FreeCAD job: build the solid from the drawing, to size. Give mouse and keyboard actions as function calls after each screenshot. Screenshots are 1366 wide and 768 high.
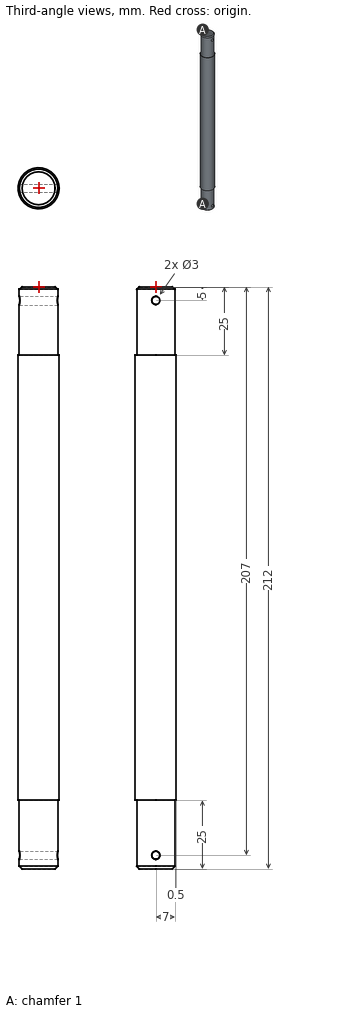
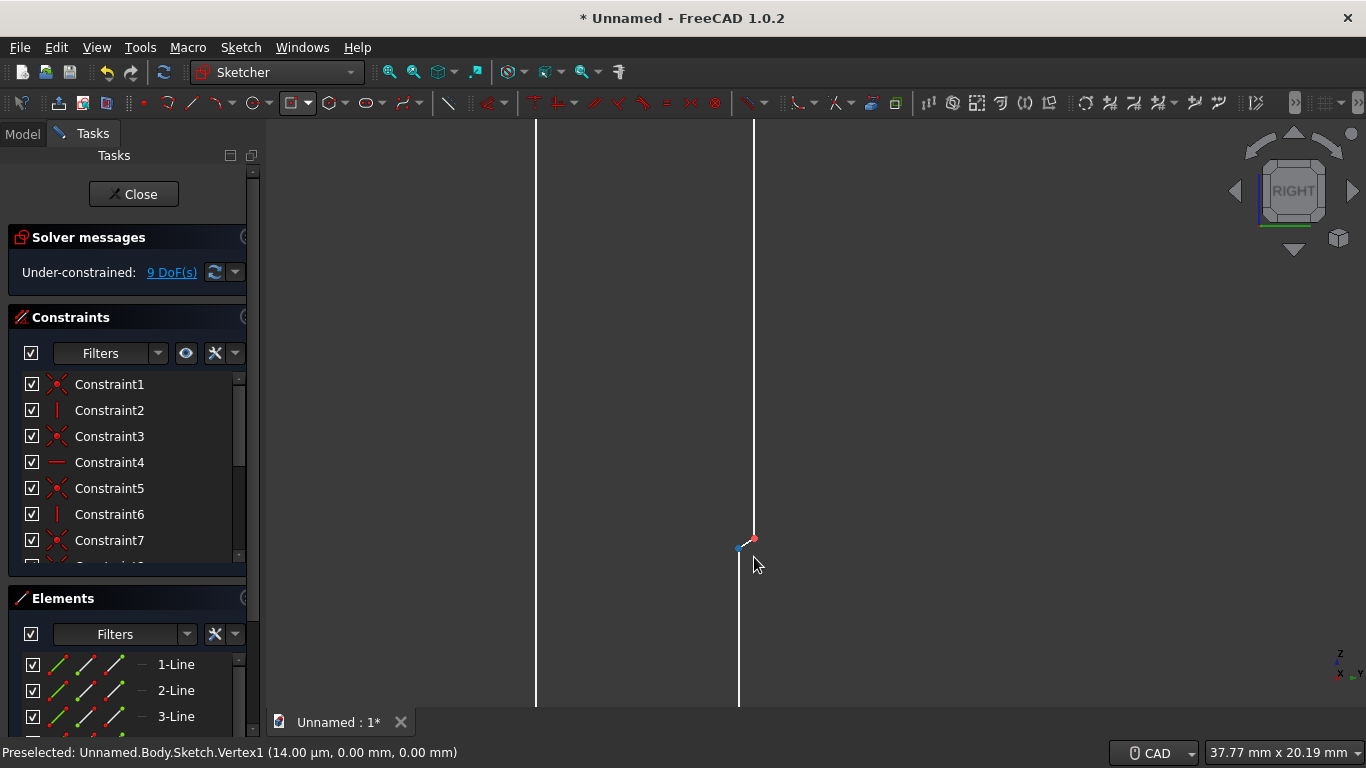
click(746, 543)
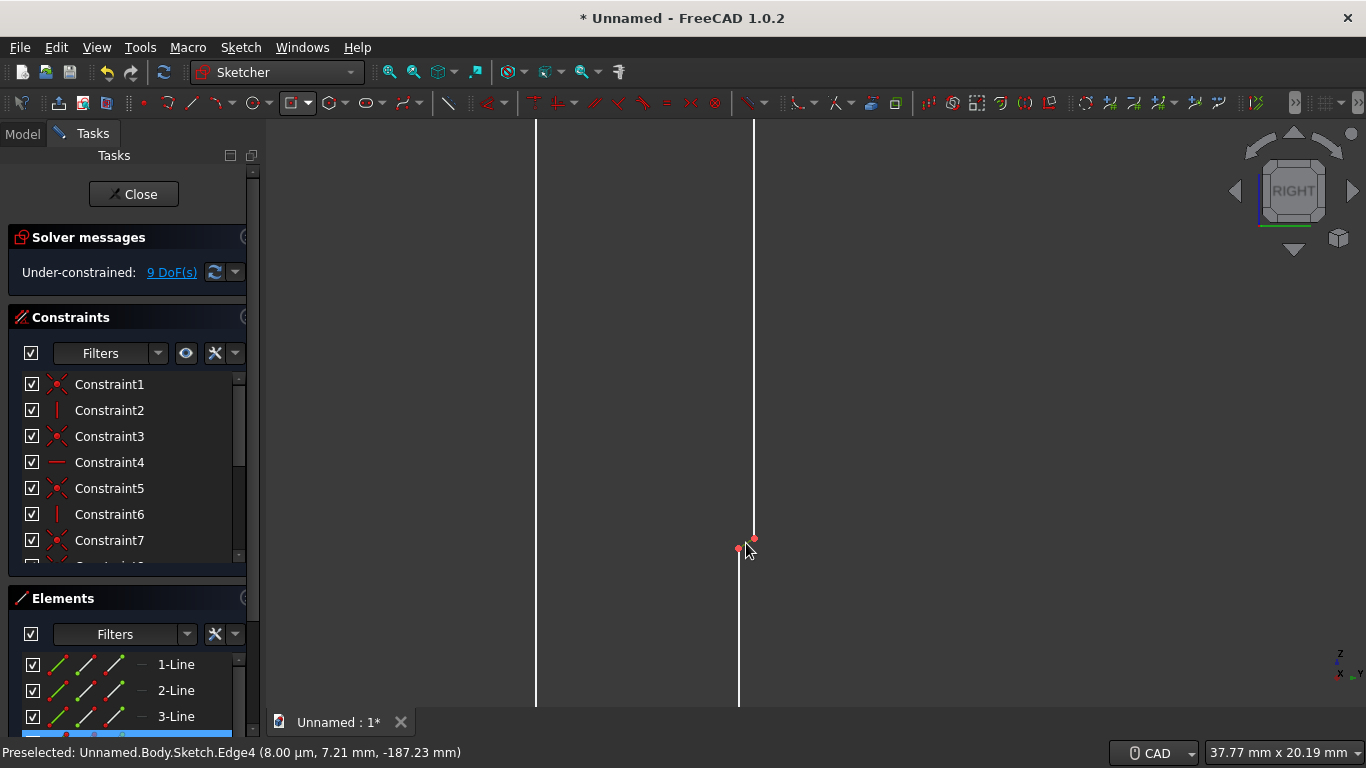
key(h)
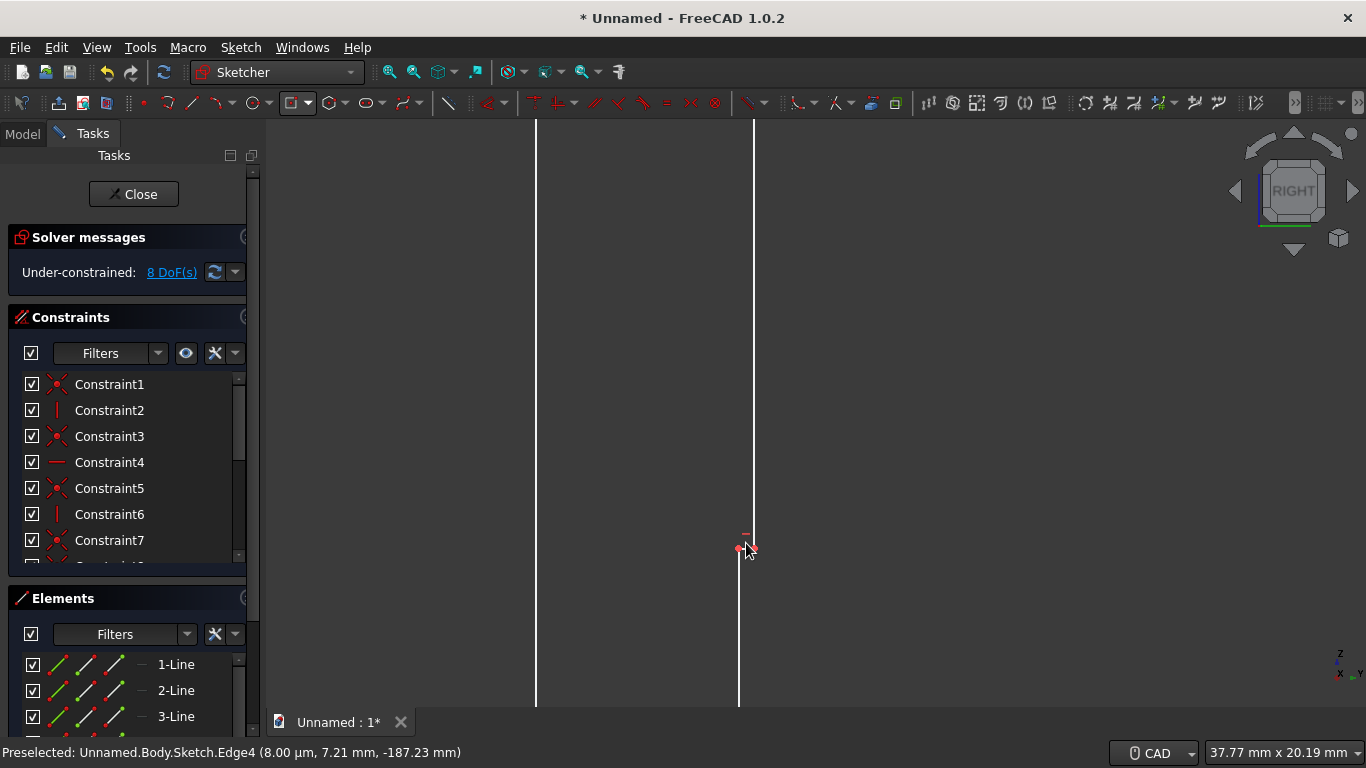
scroll(754, 558, down, 14)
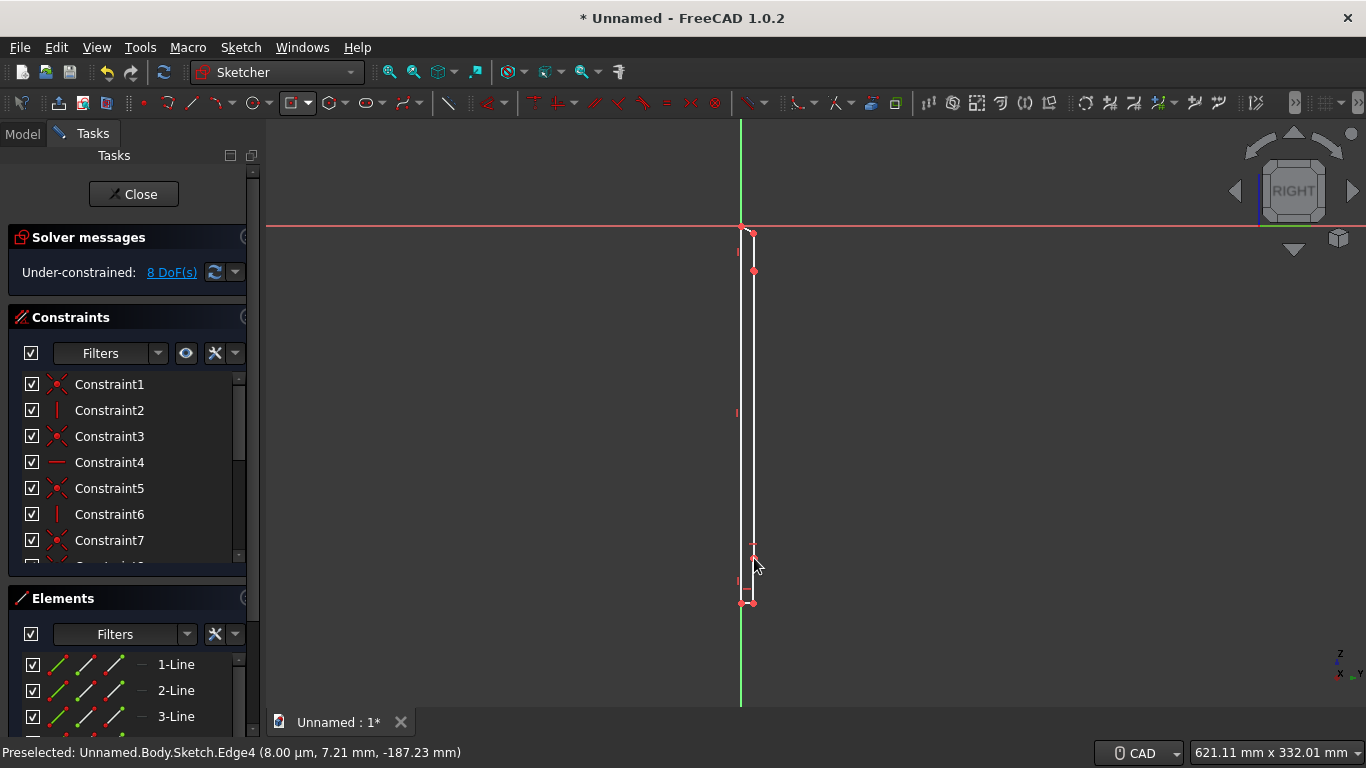
scroll(754, 271, up, 14)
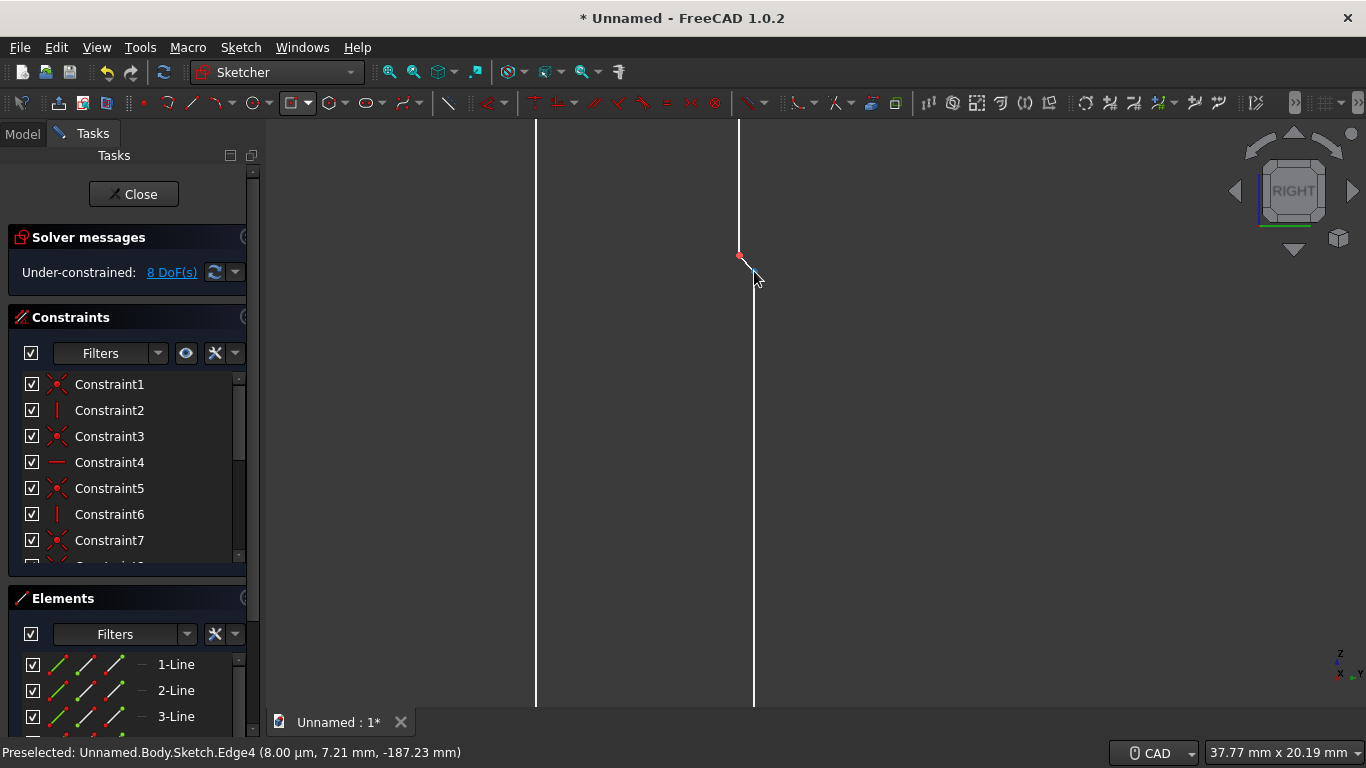
click(747, 264)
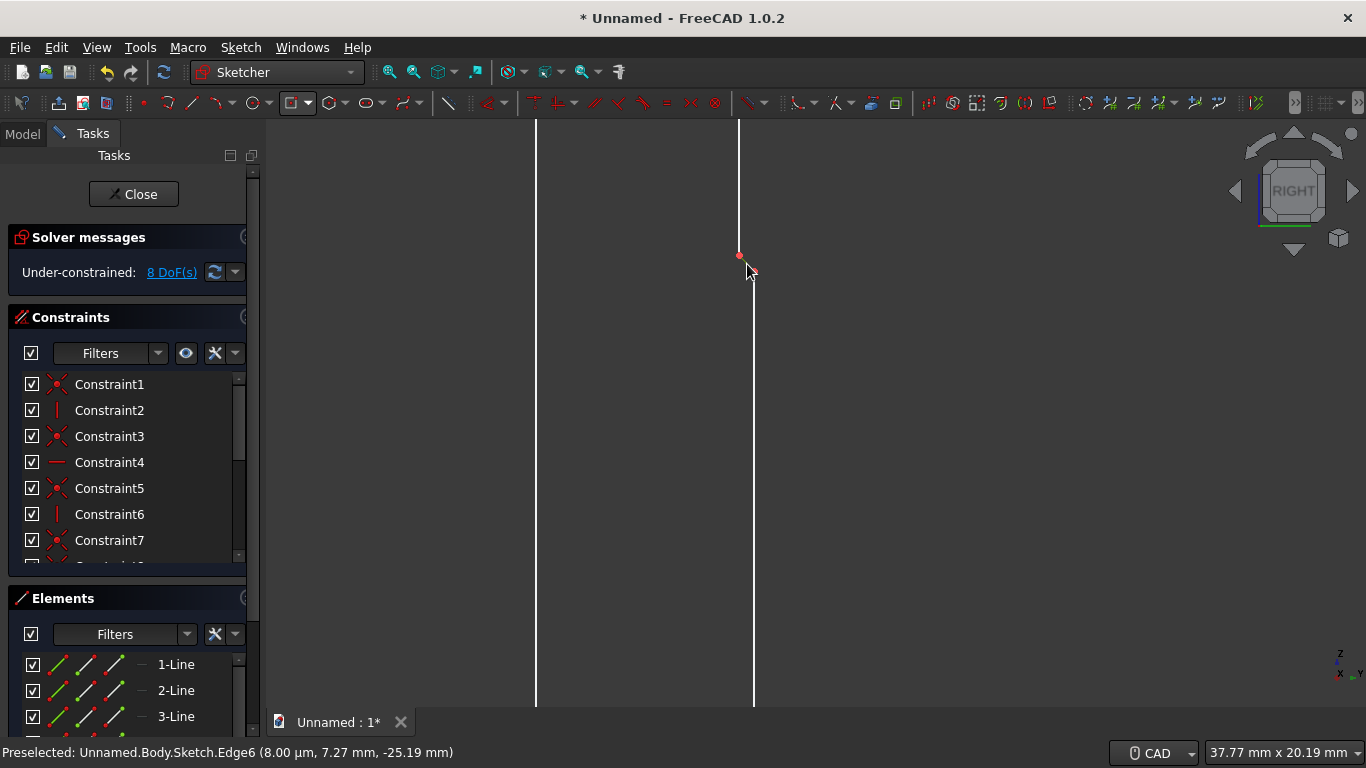
key(h)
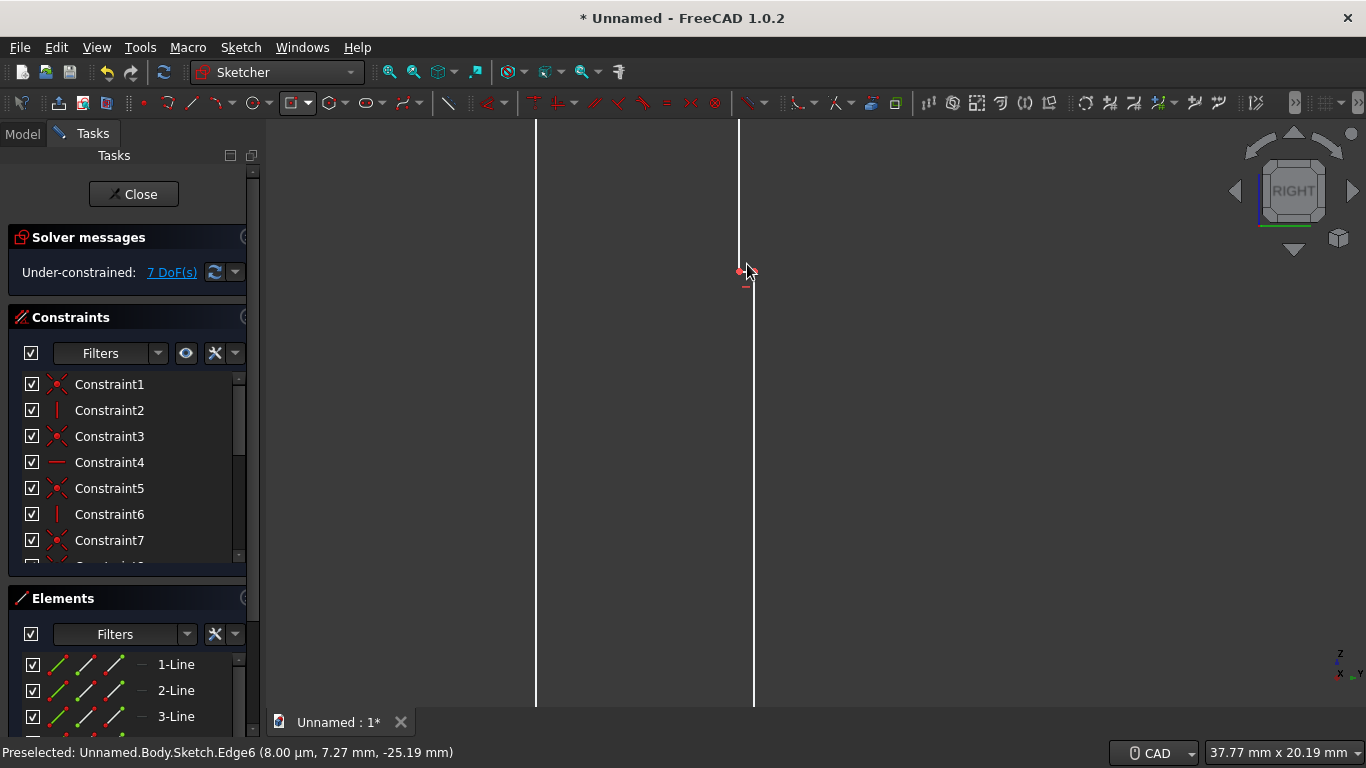
scroll(754, 270, down, 14)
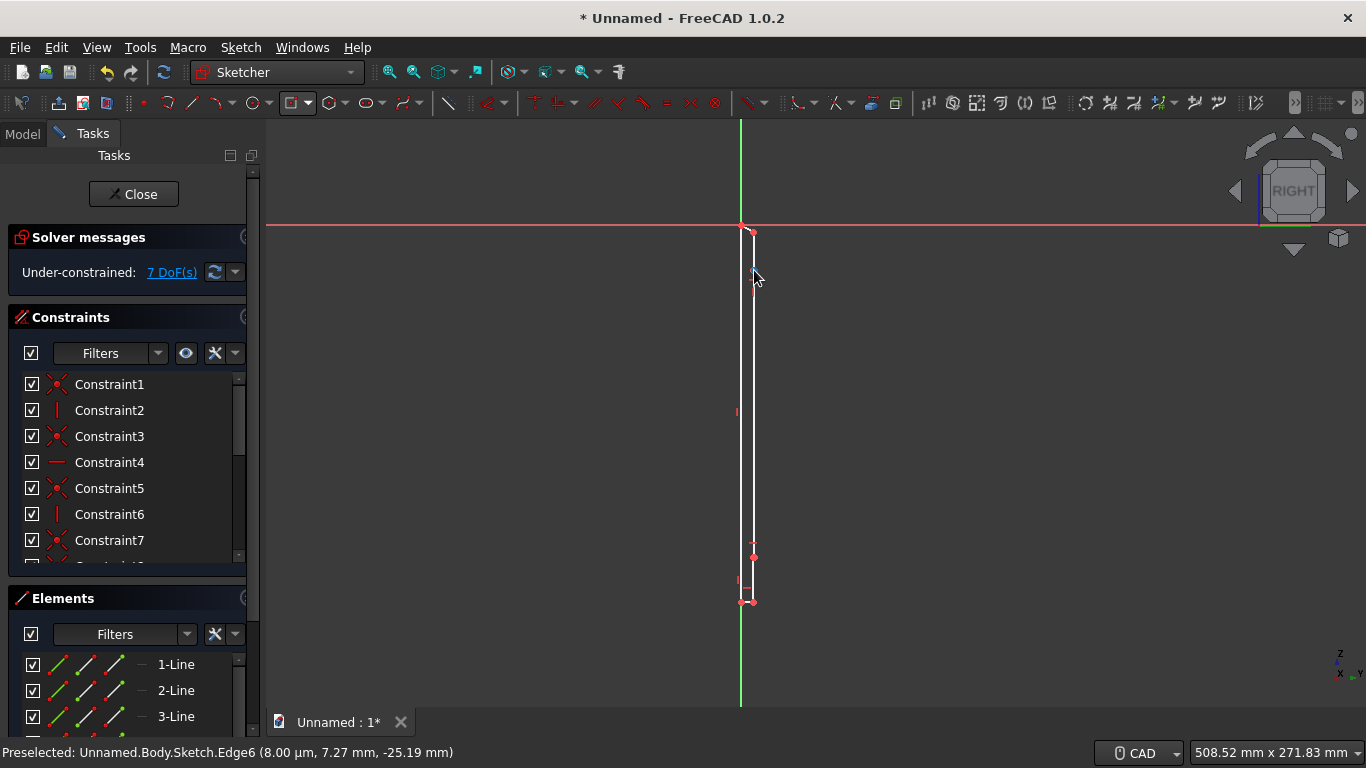
scroll(750, 230, up, 6)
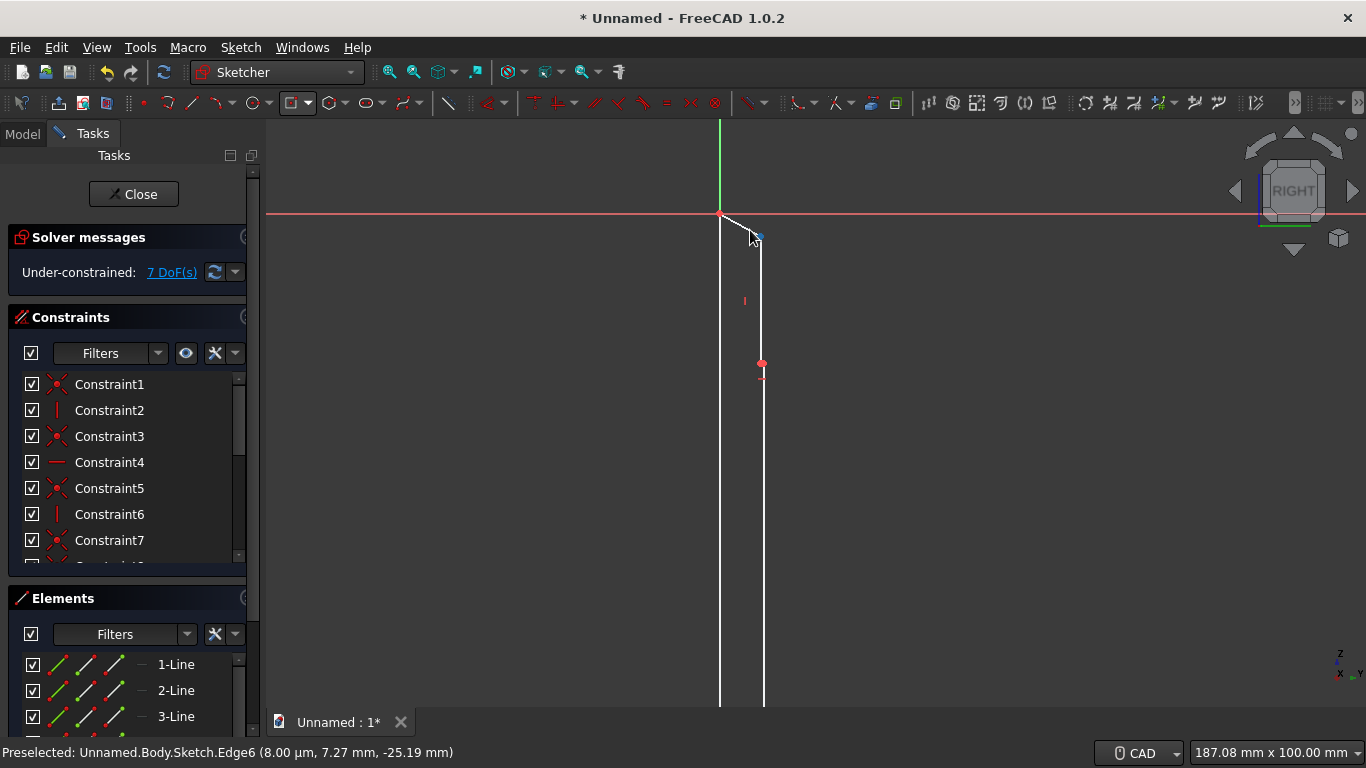
click(748, 230)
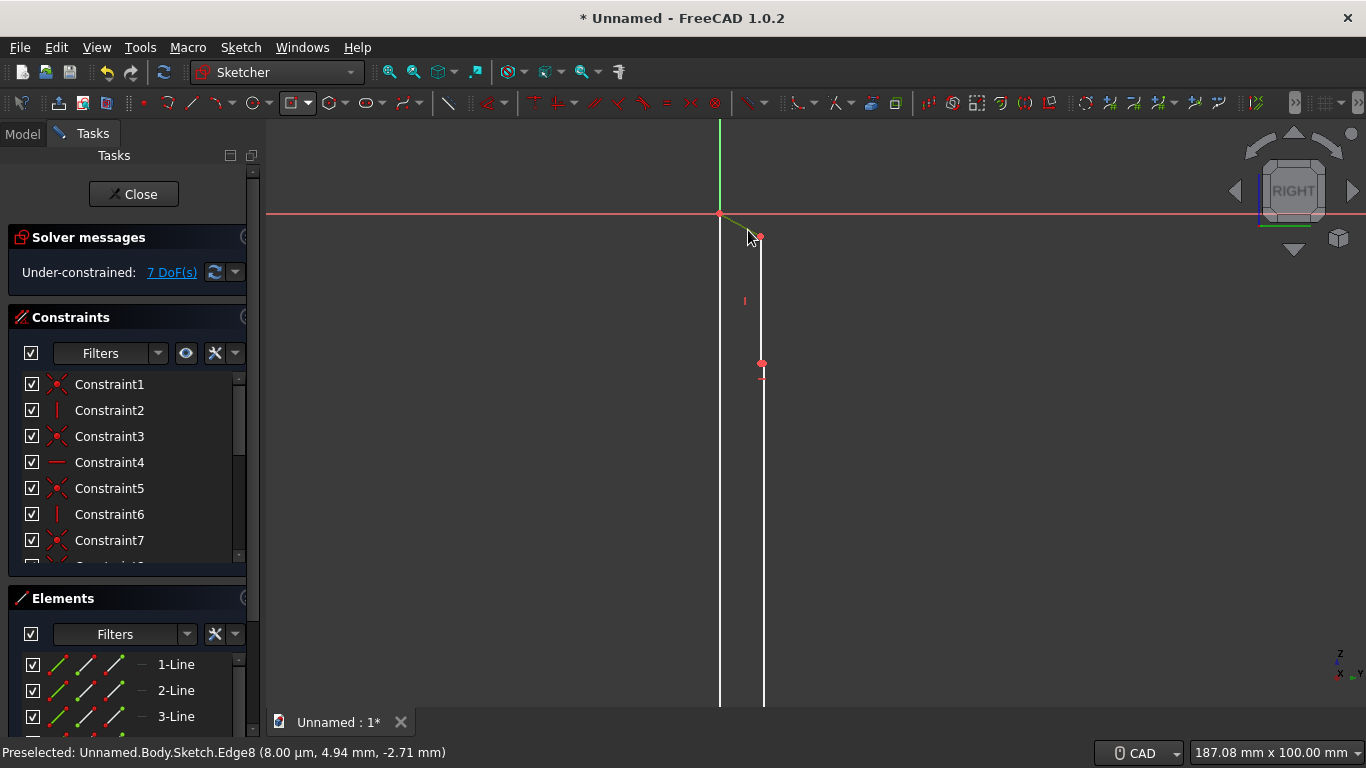
click(576, 104)